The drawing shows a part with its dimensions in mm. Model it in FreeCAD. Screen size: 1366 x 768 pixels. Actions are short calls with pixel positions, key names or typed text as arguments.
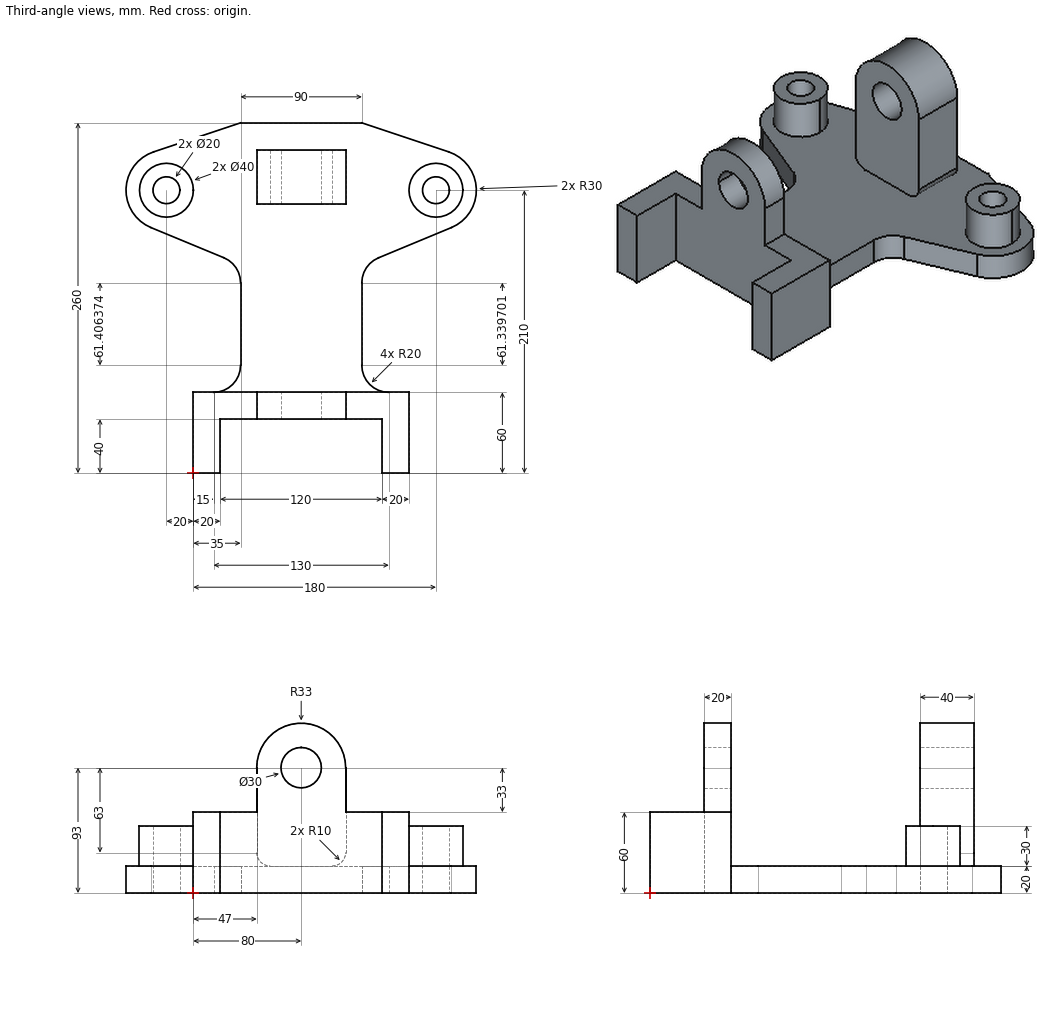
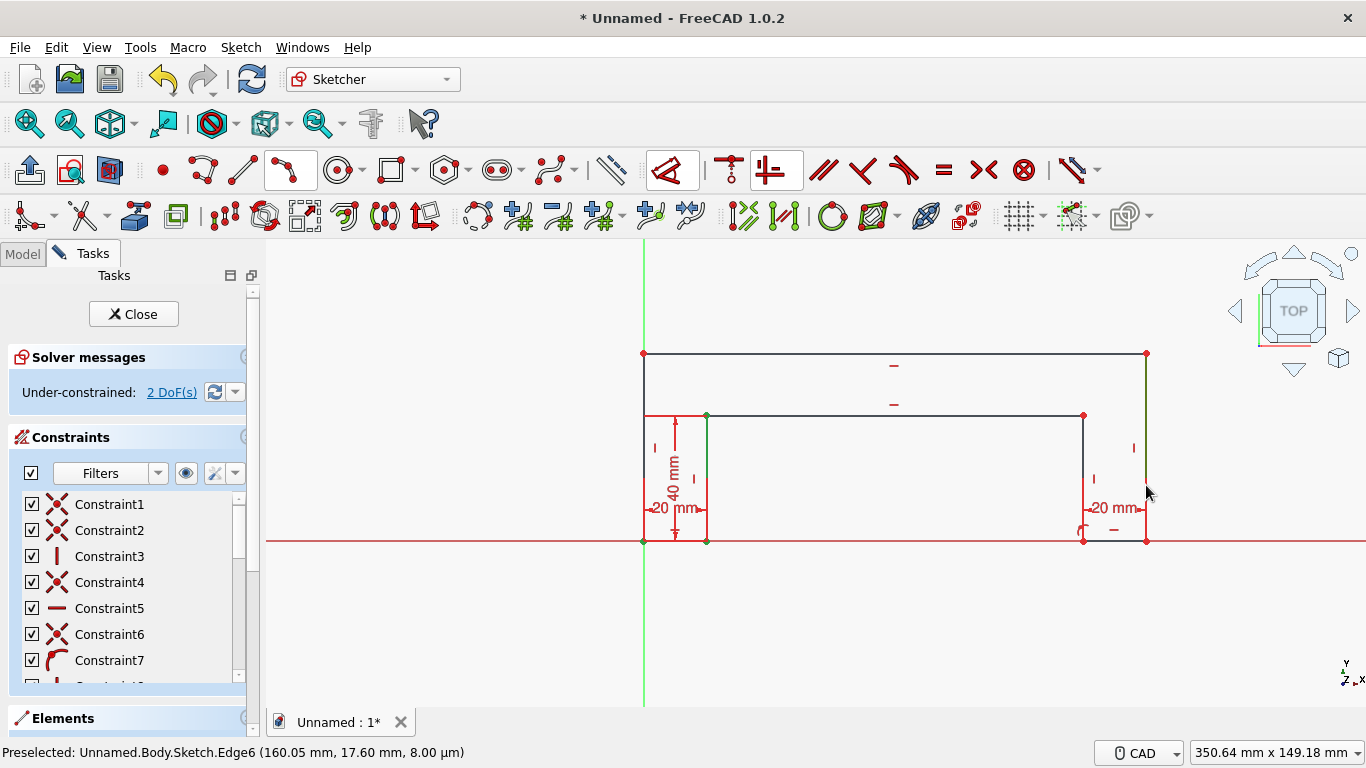
key(i)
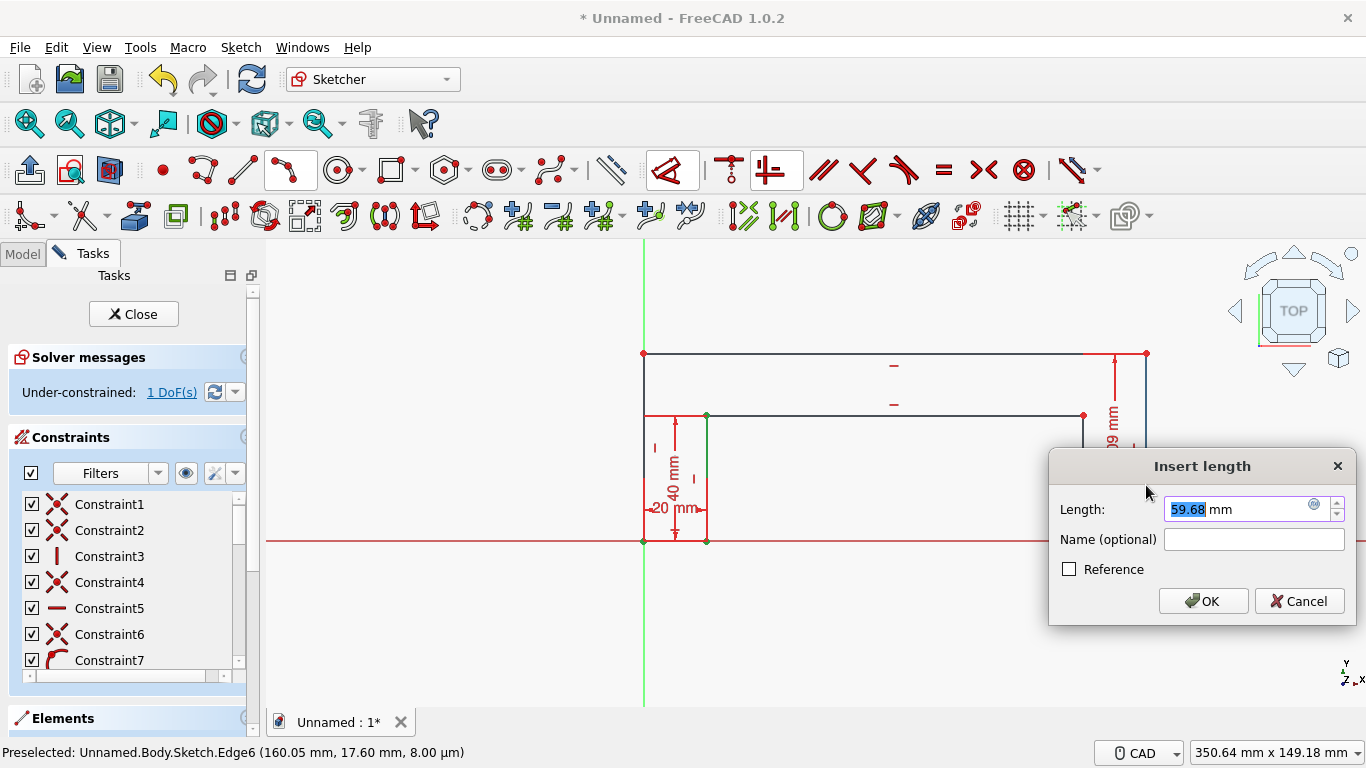
text(60)
key(Return)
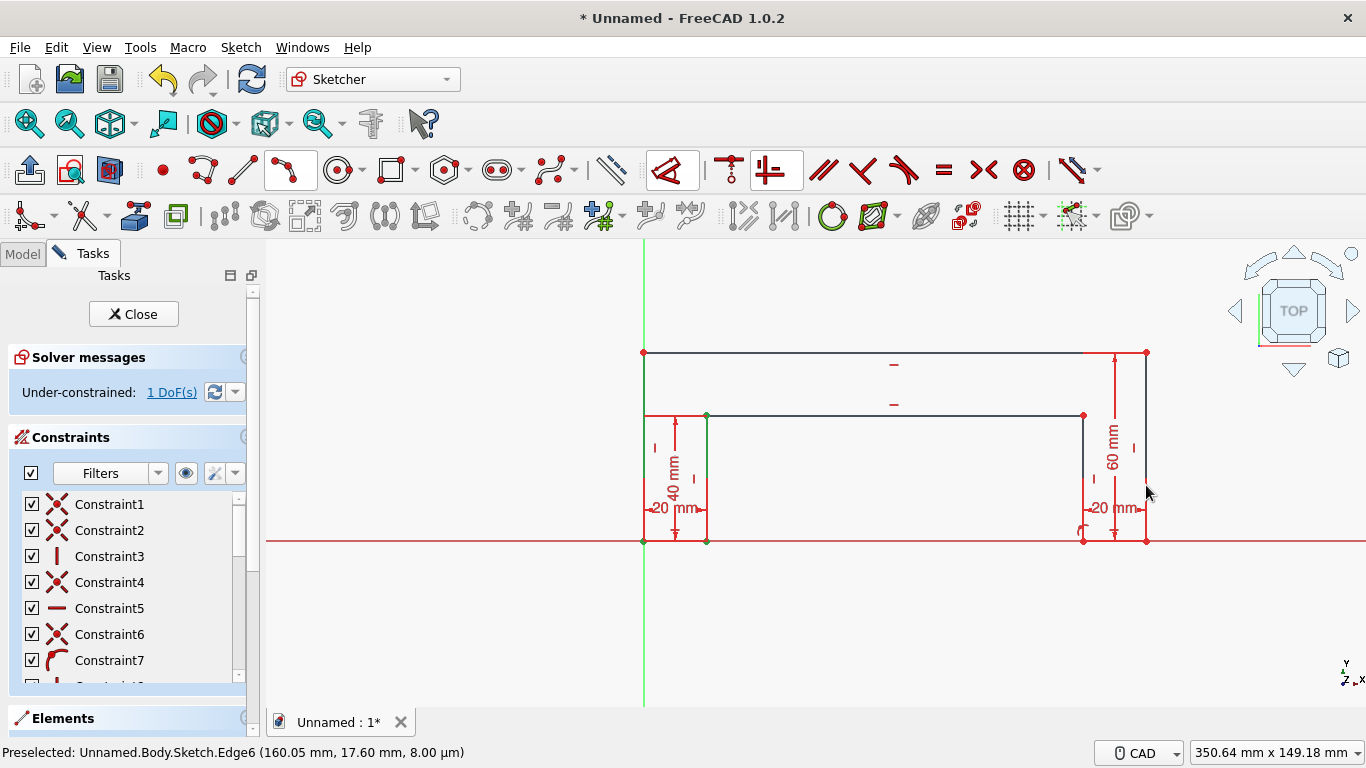
click(820, 416)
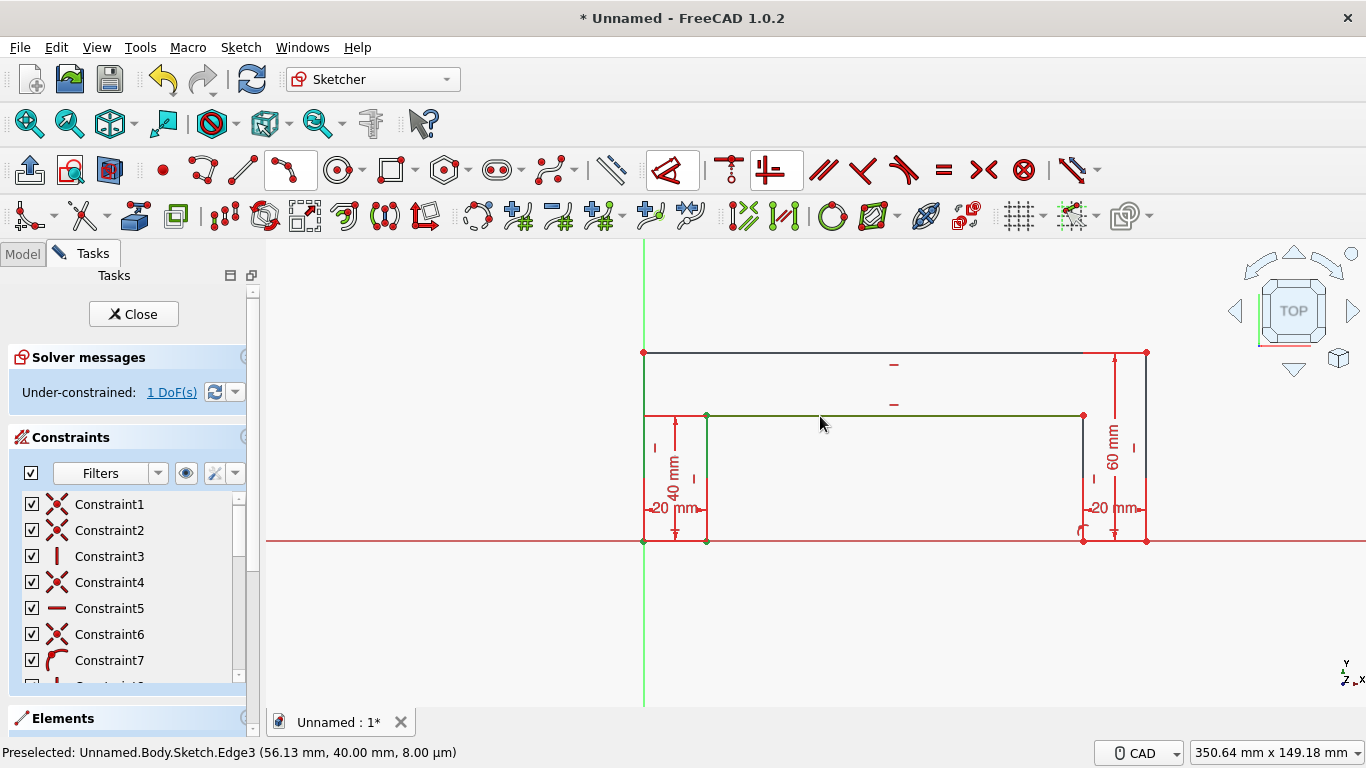
key(l)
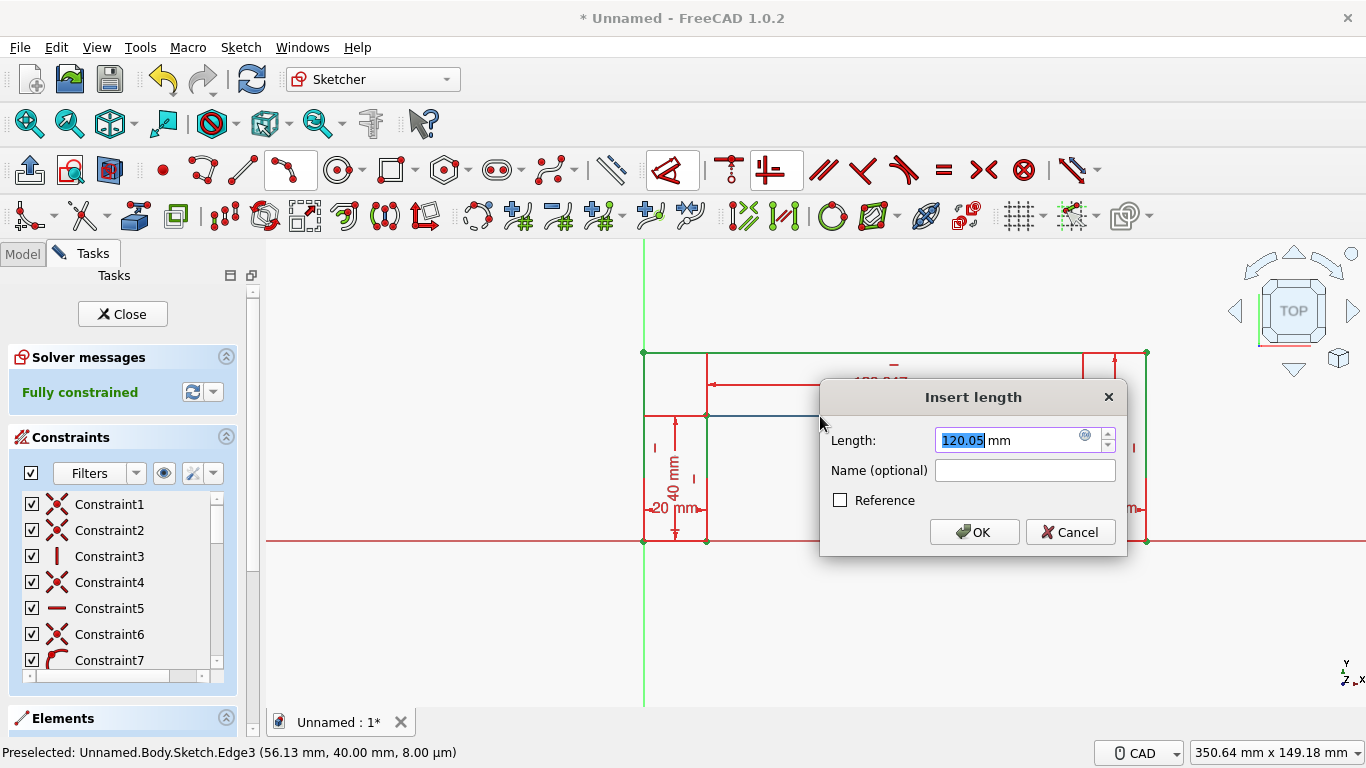
text(120)
key(Return)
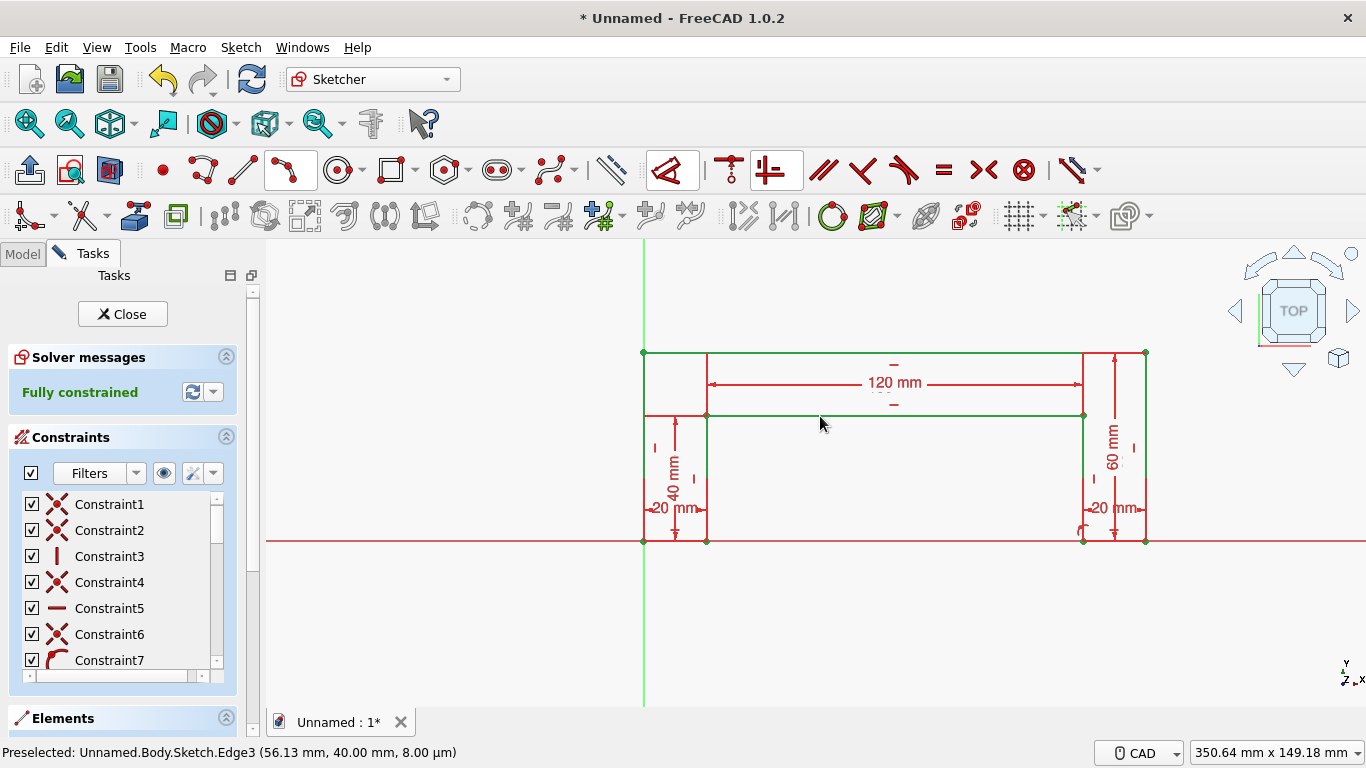
click(123, 314)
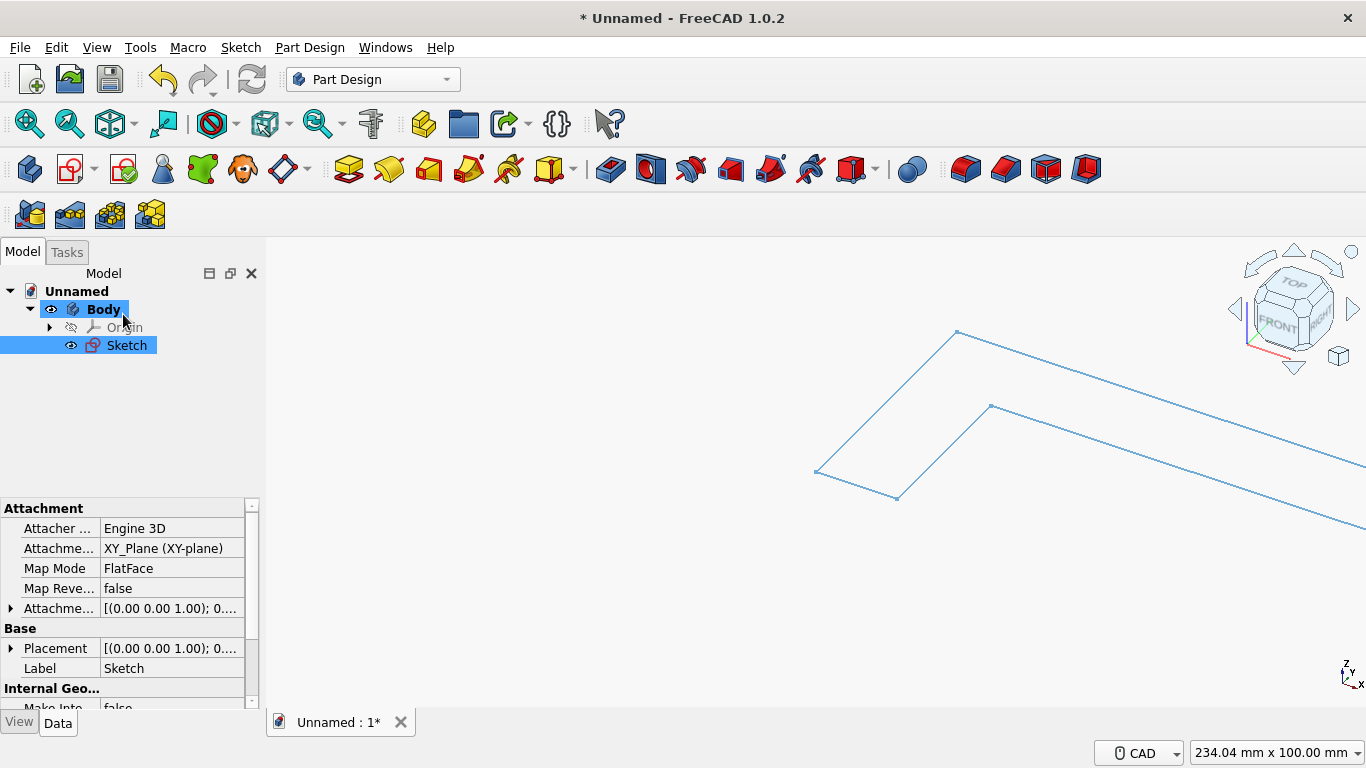
click(350, 170)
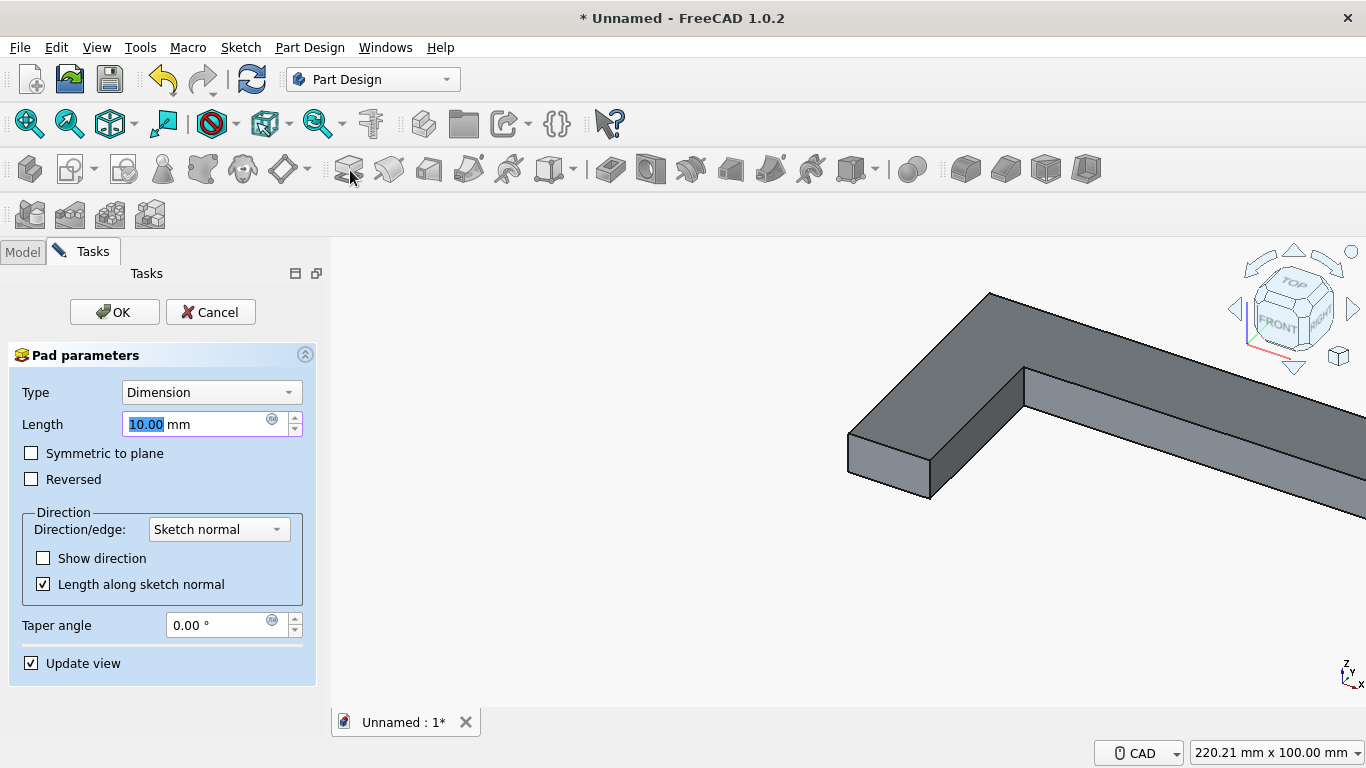
text(60)
key(Tab)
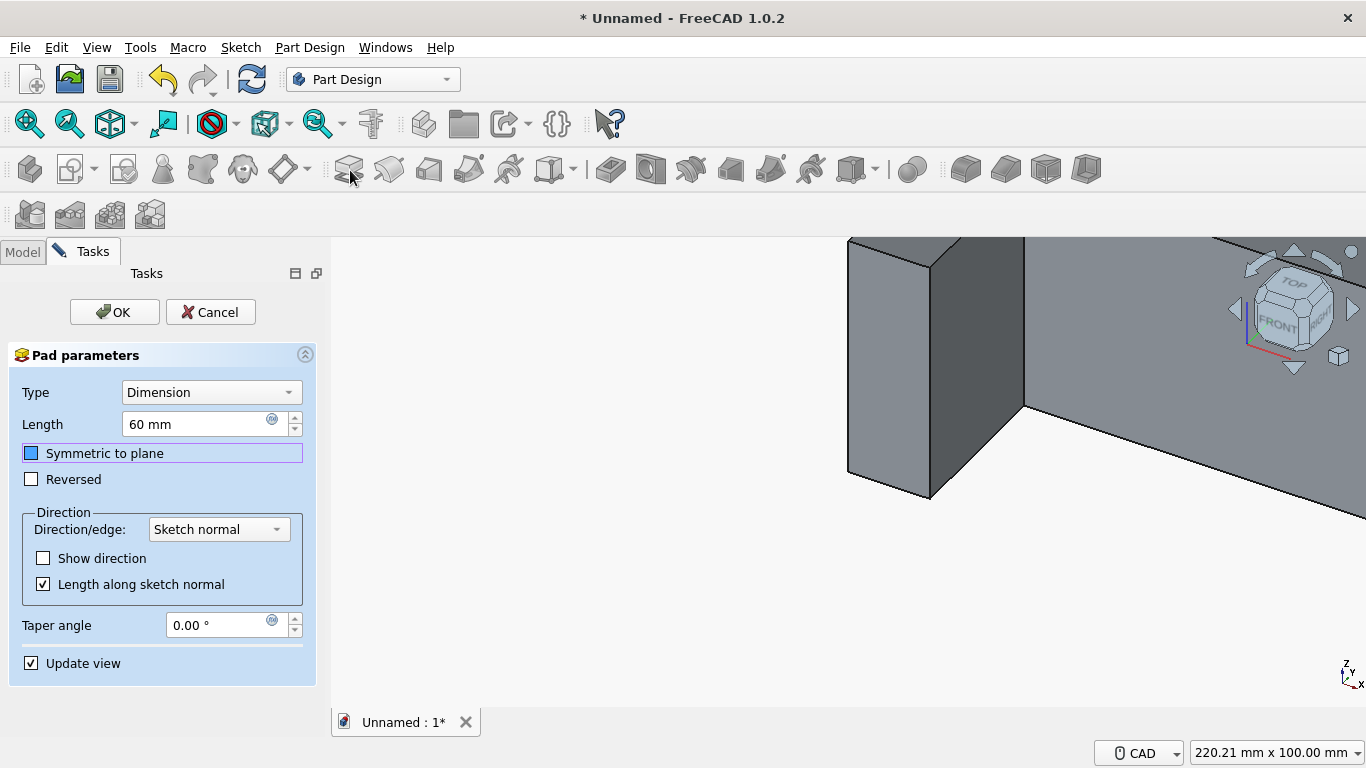
click(115, 312)